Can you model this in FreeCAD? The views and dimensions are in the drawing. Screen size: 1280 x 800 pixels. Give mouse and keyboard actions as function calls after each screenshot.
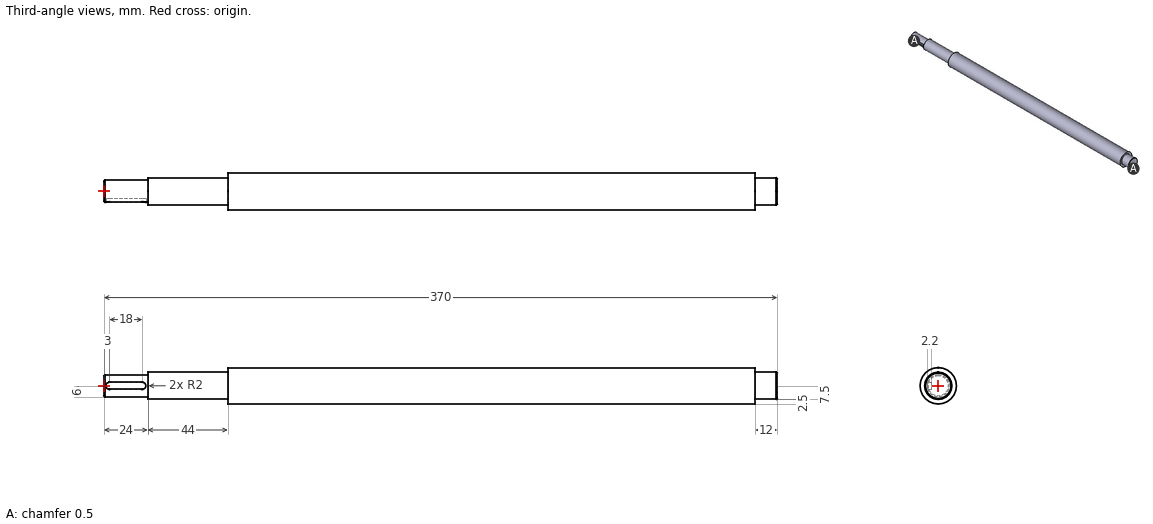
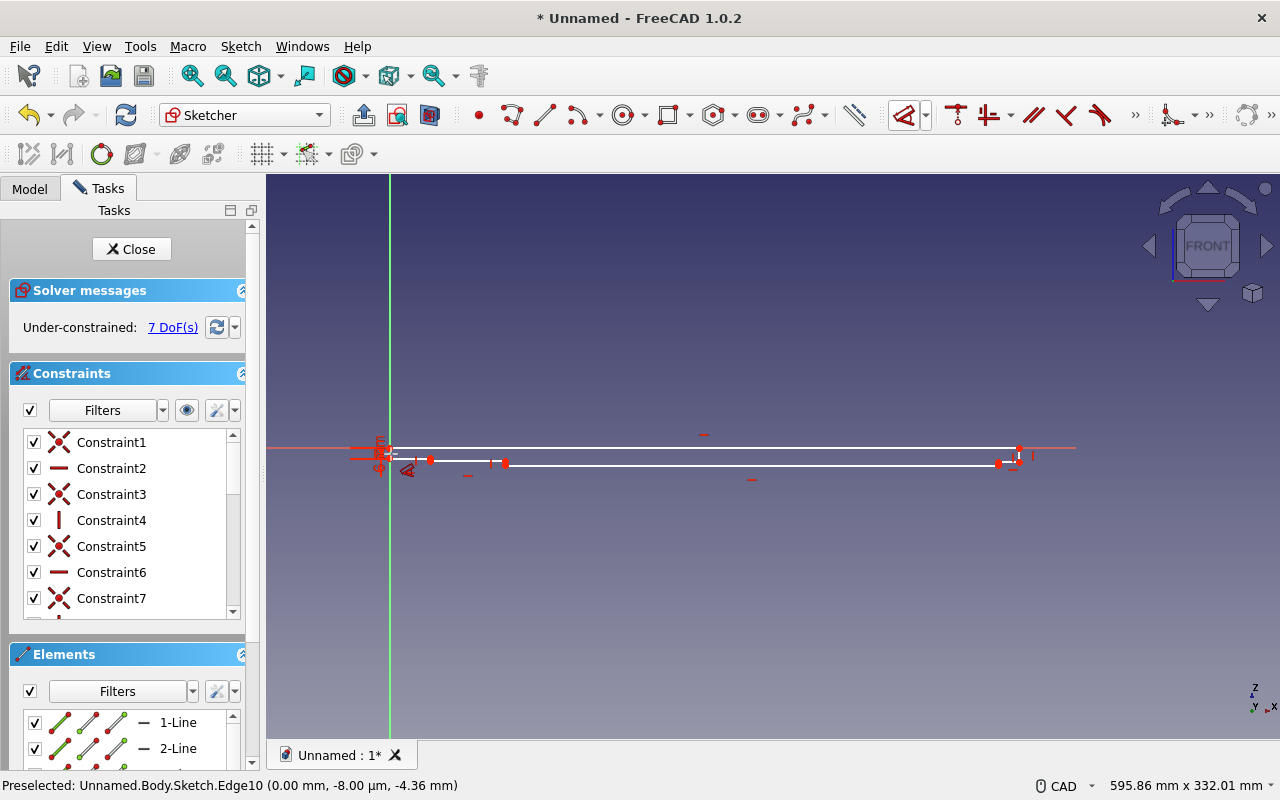
scroll(1013, 462, up, 5)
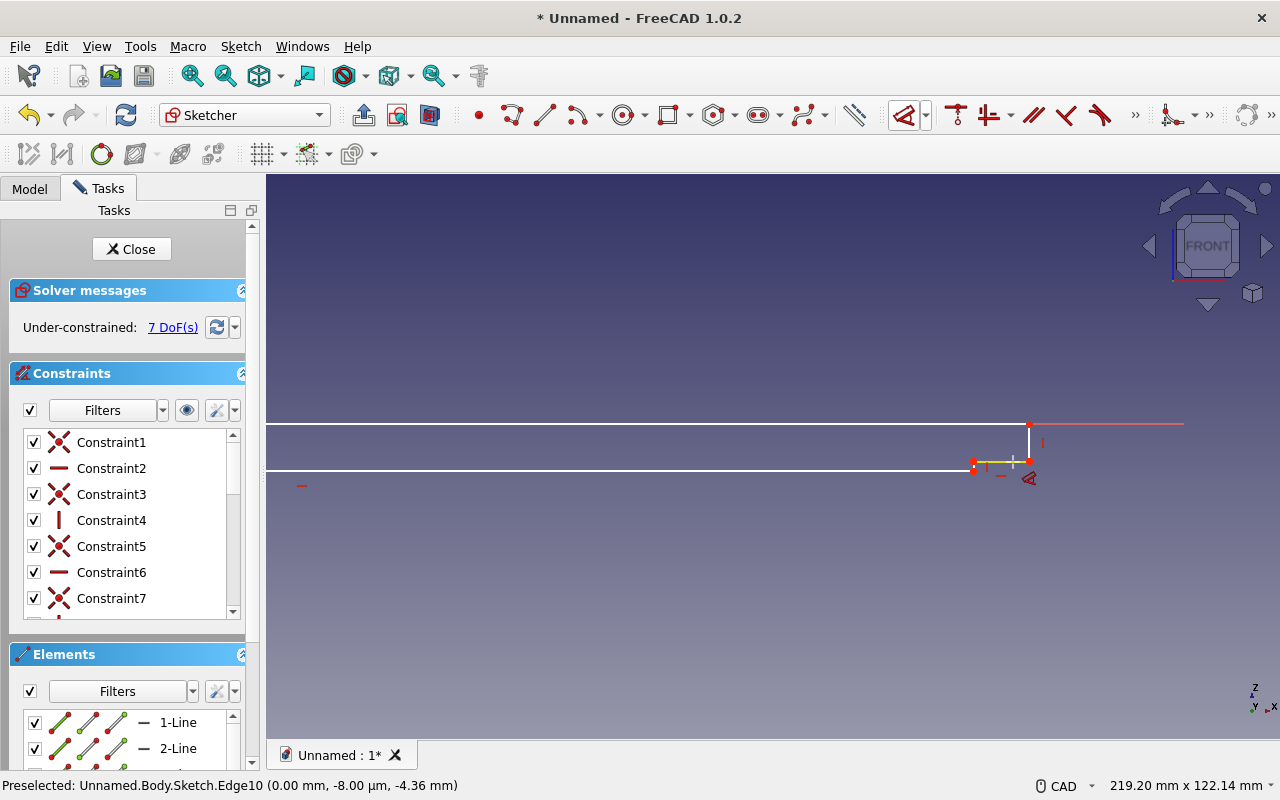
click(1013, 462)
click(1001, 496)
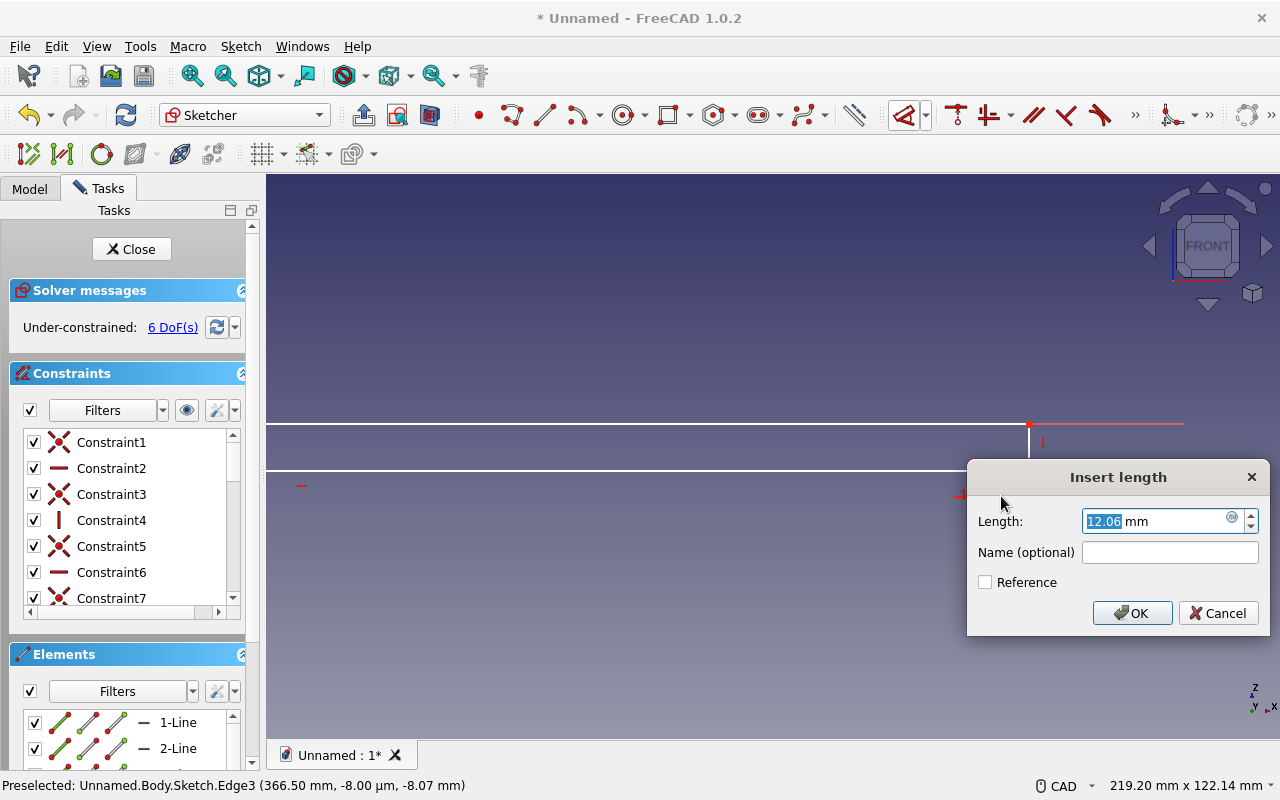
text(12)
key(Return)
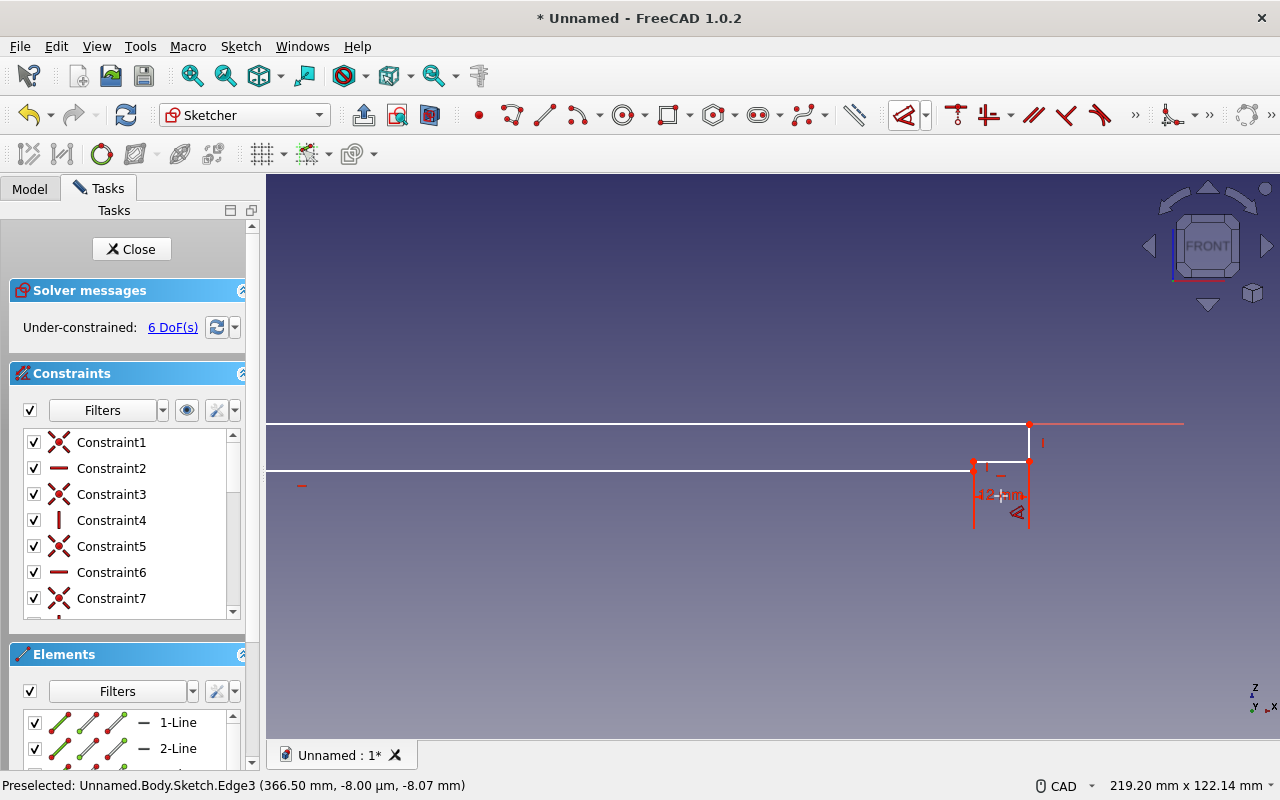
scroll(1014, 462, down, 5)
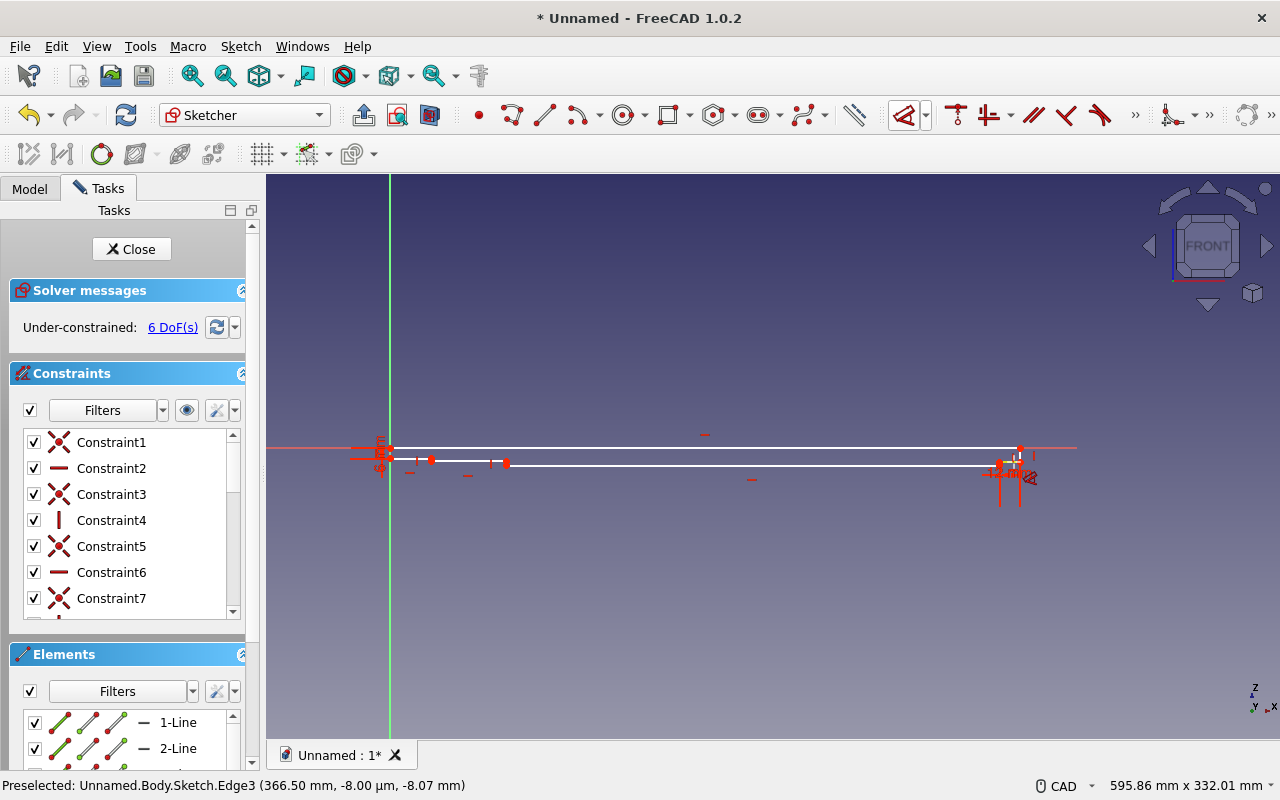
click(484, 461)
click(469, 495)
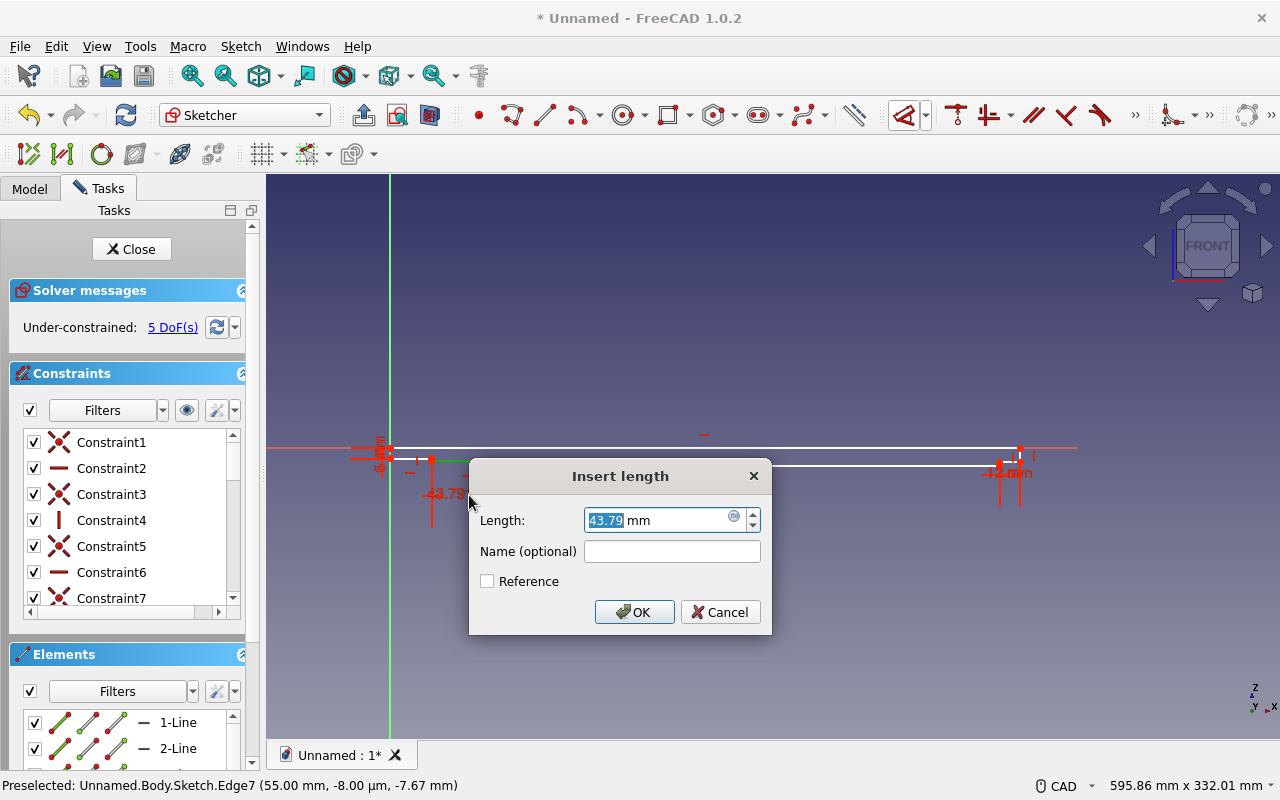
text(44)
key(Return)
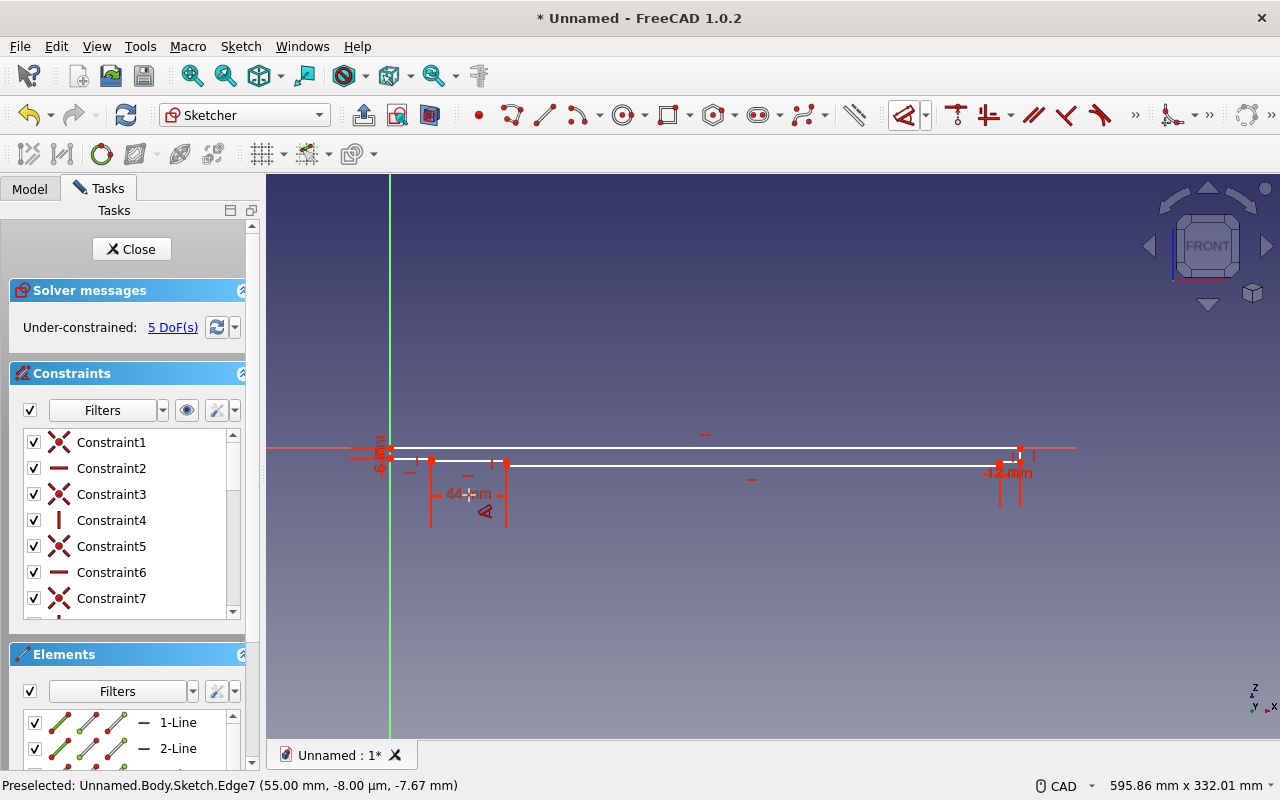
scroll(419, 459, up, 2)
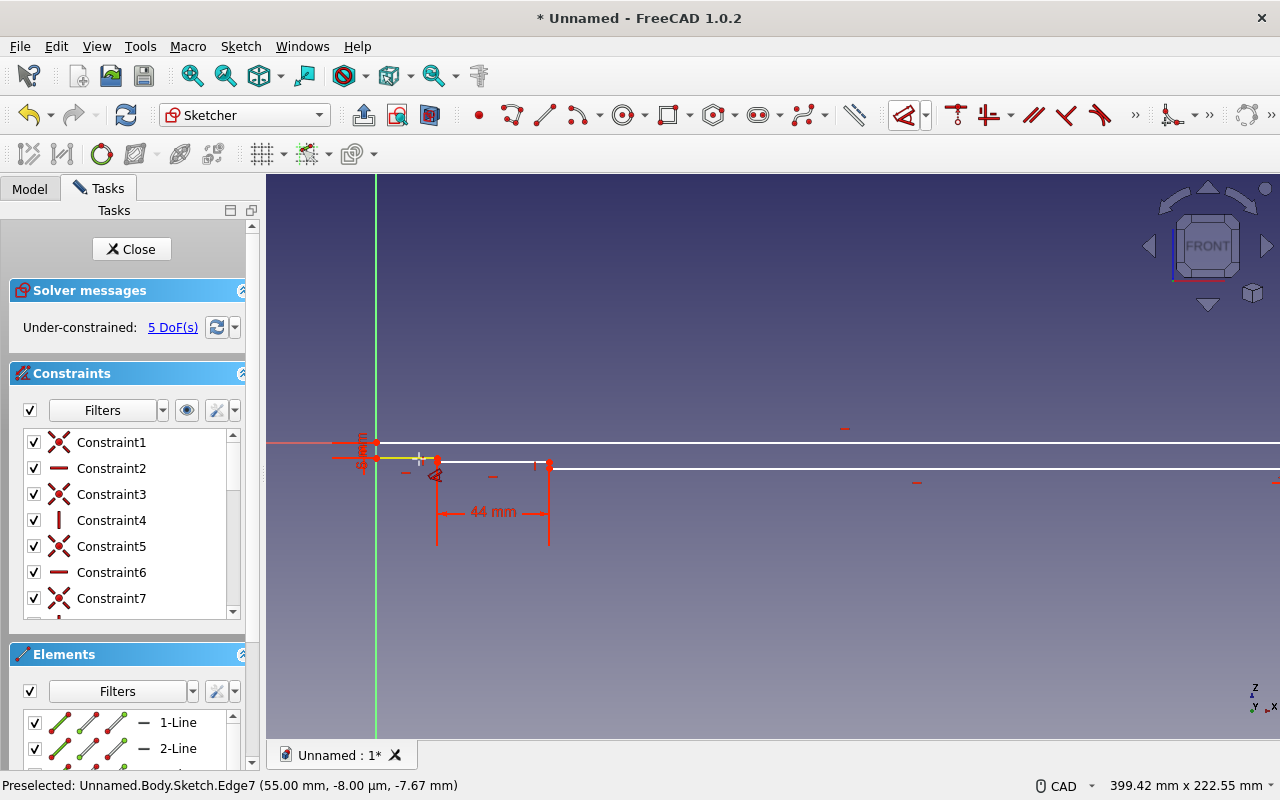
click(419, 458)
click(407, 492)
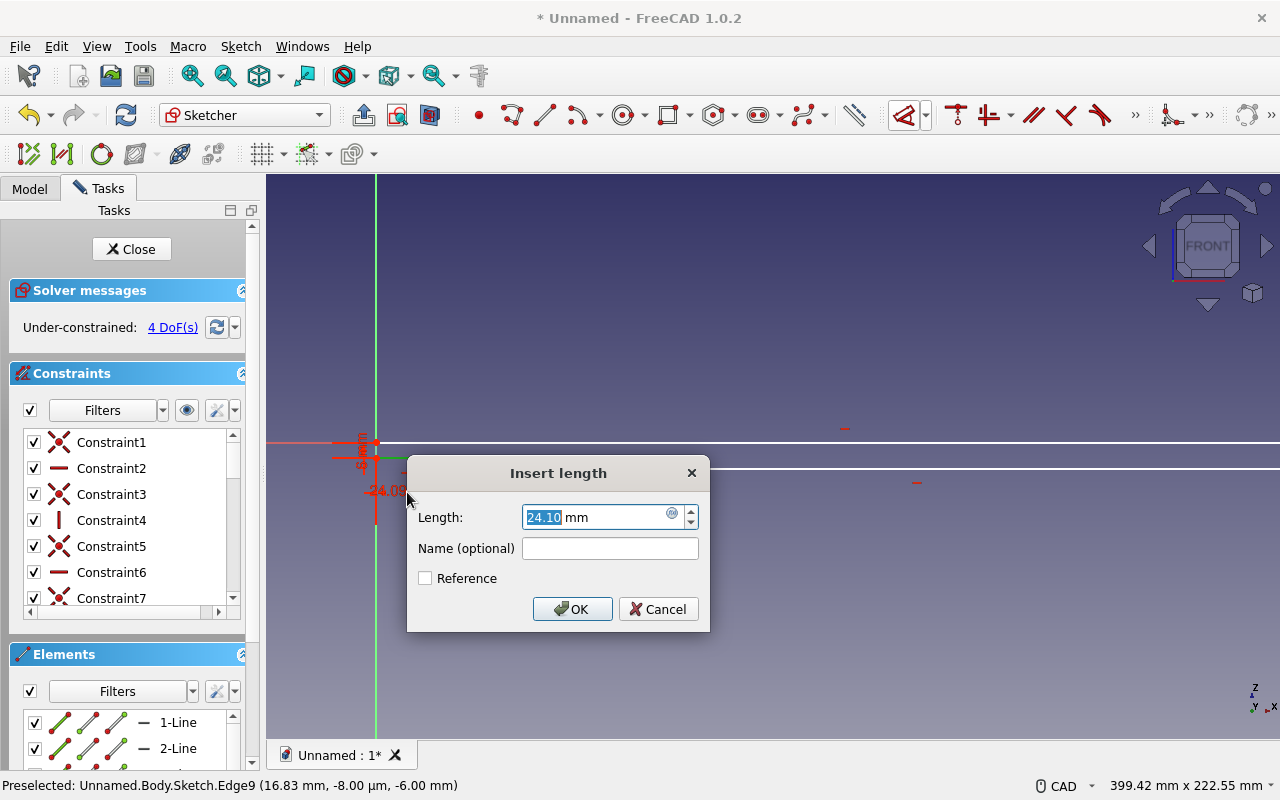
text(24)
key(Return)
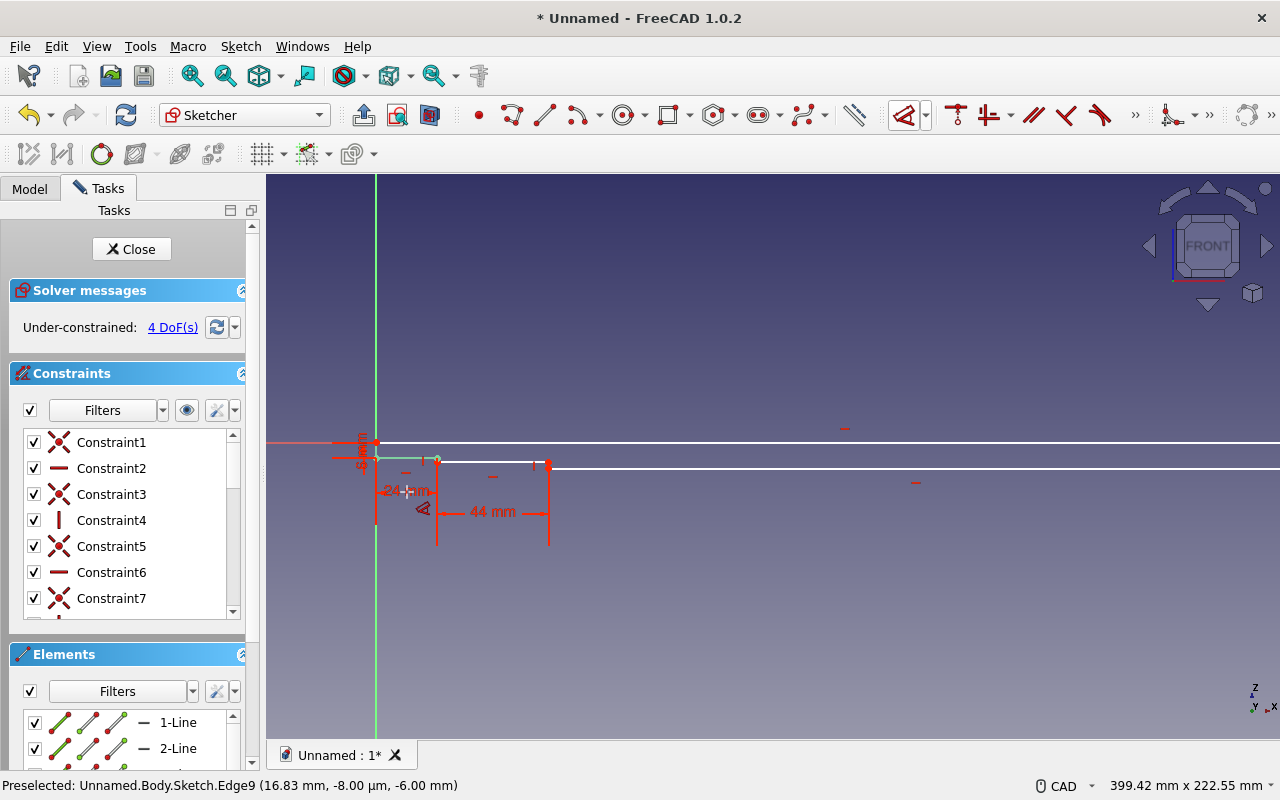
click(658, 443)
click(746, 409)